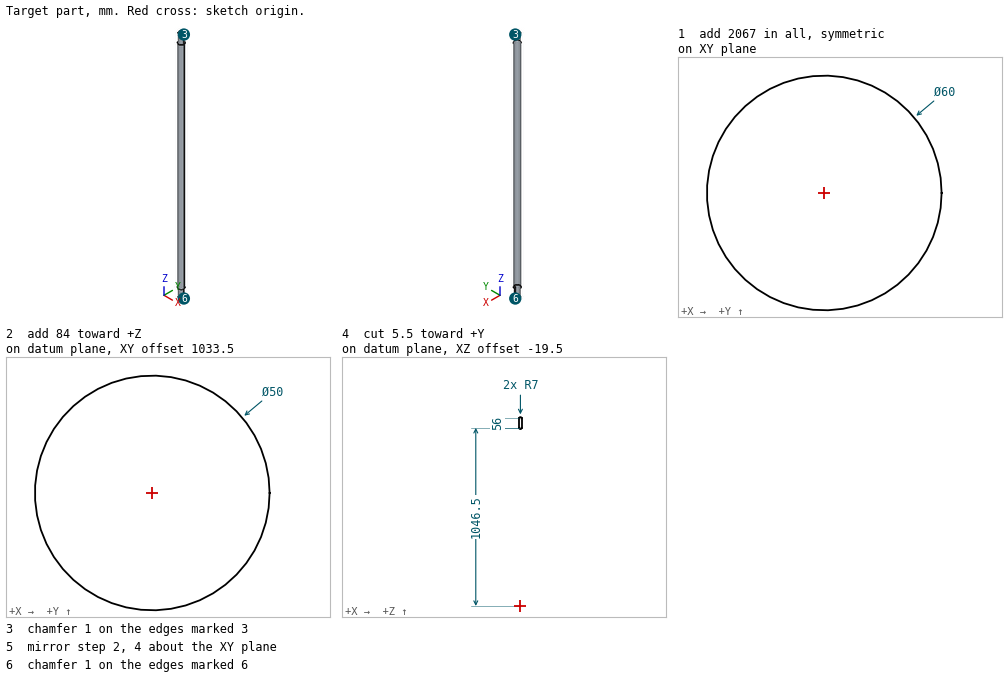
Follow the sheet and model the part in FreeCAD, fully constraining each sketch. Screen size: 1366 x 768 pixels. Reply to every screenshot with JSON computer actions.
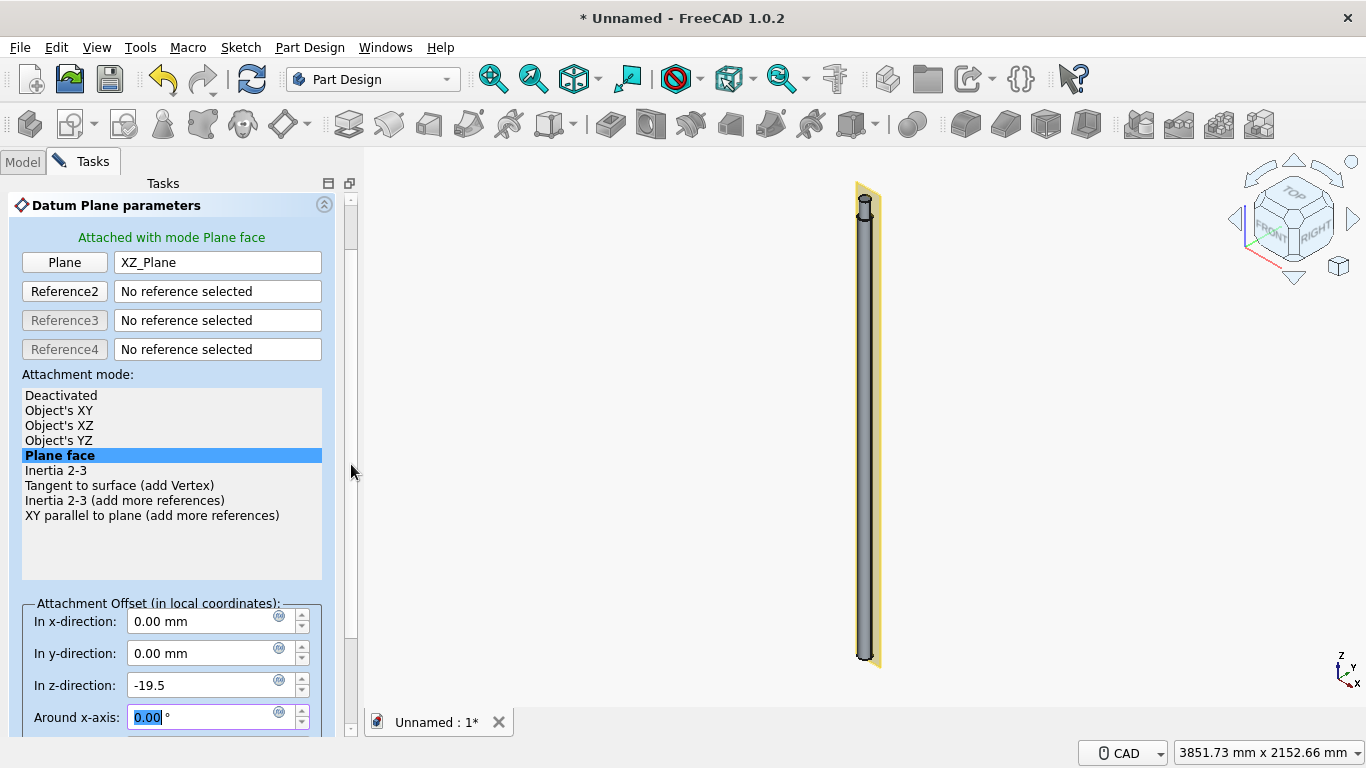
{"action": "left_click", "coordinate": [124, 222]}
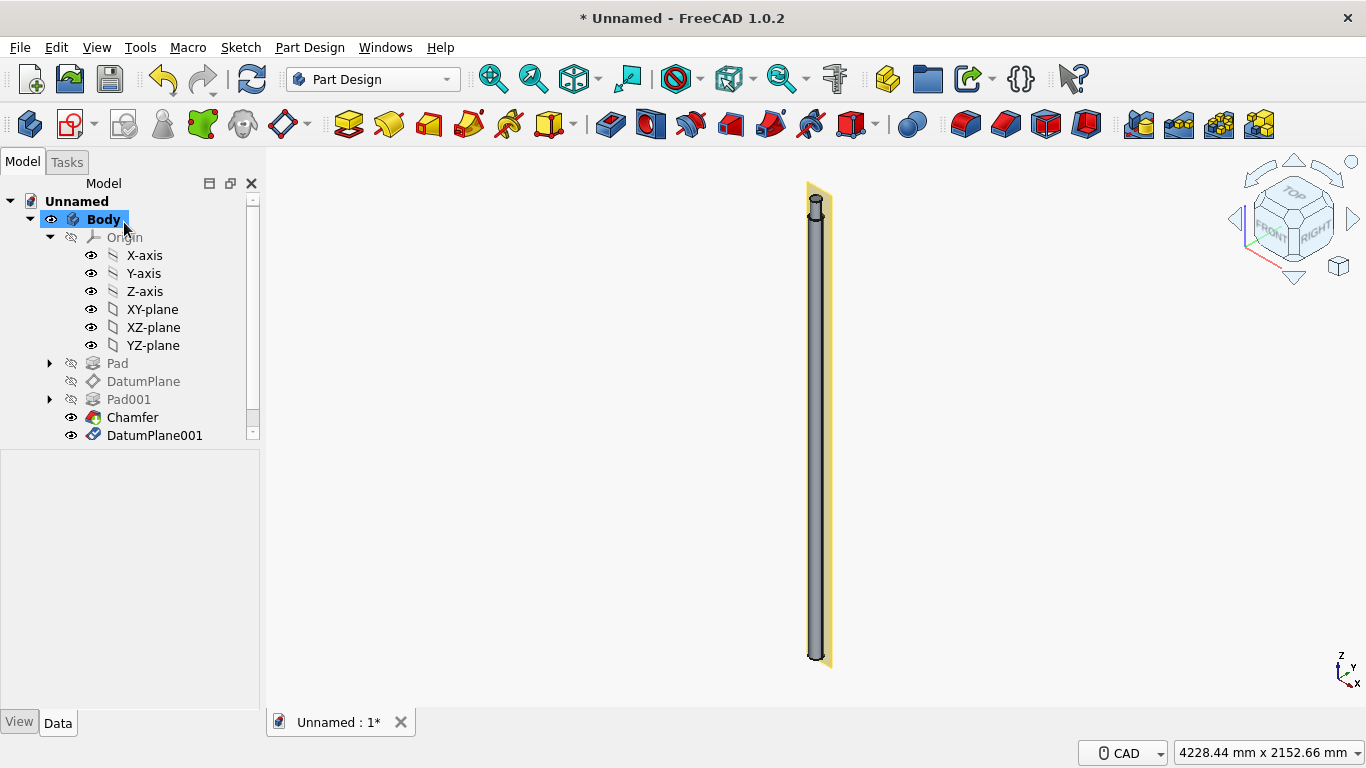
{"action": "left_click", "coordinate": [116, 435]}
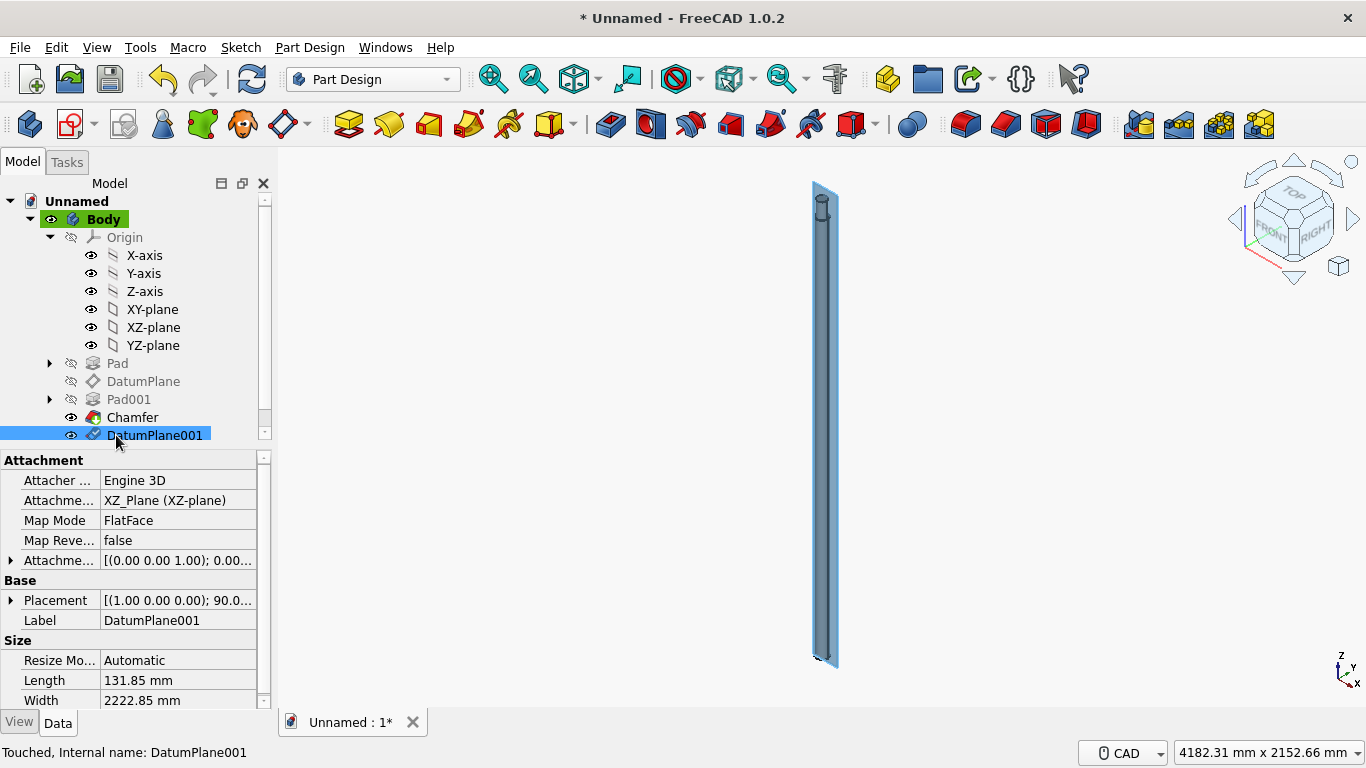
{"action": "left_click", "coordinate": [70, 124]}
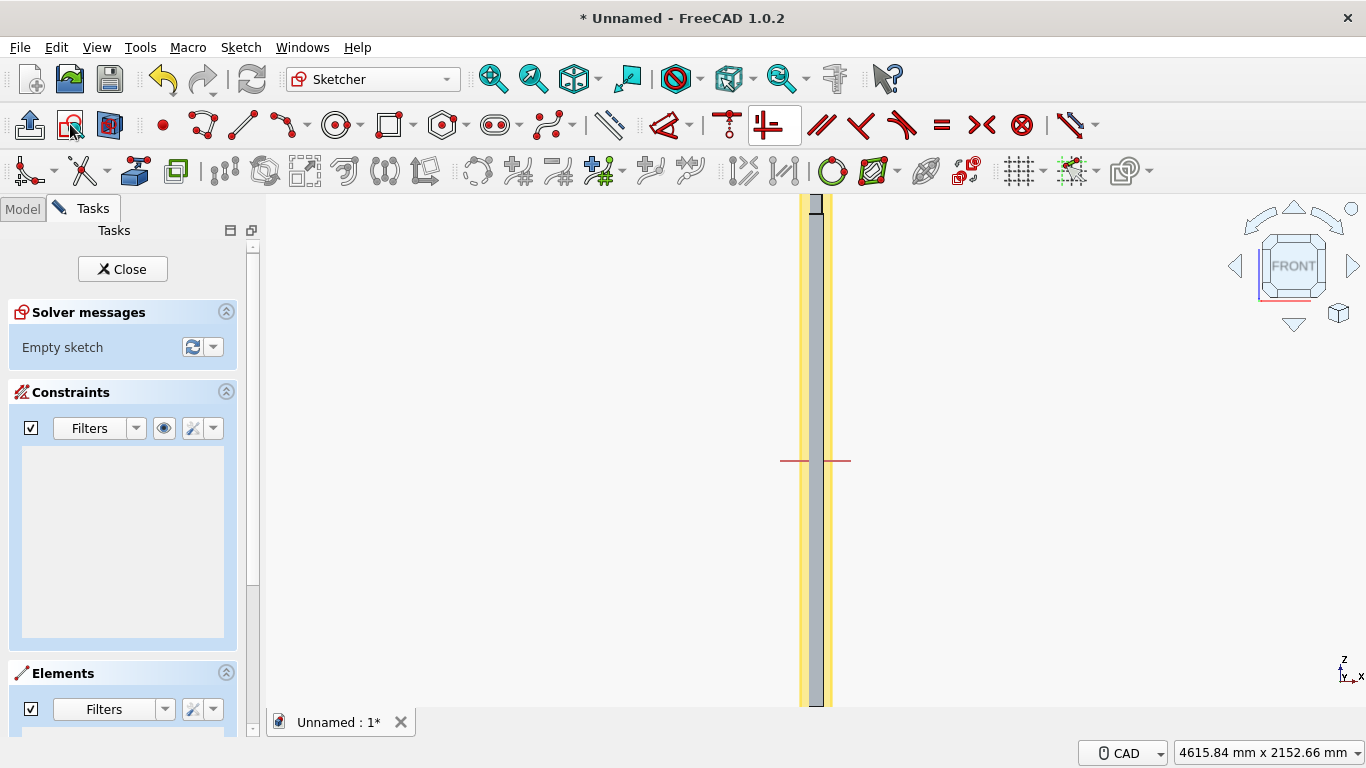
{"action": "left_click", "coordinate": [110, 126]}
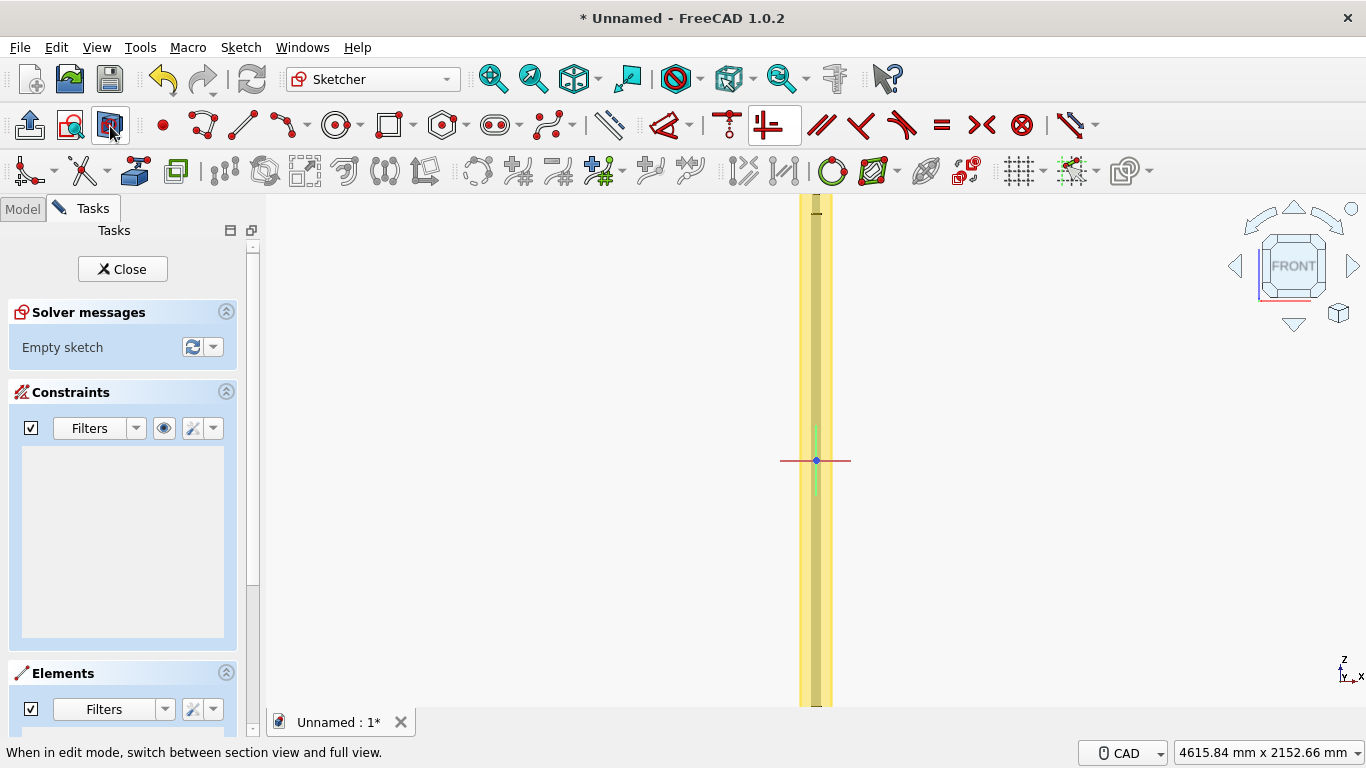
{"action": "scroll", "coordinate": [748, 450], "scroll_direction": "down", "scroll_amount": 5}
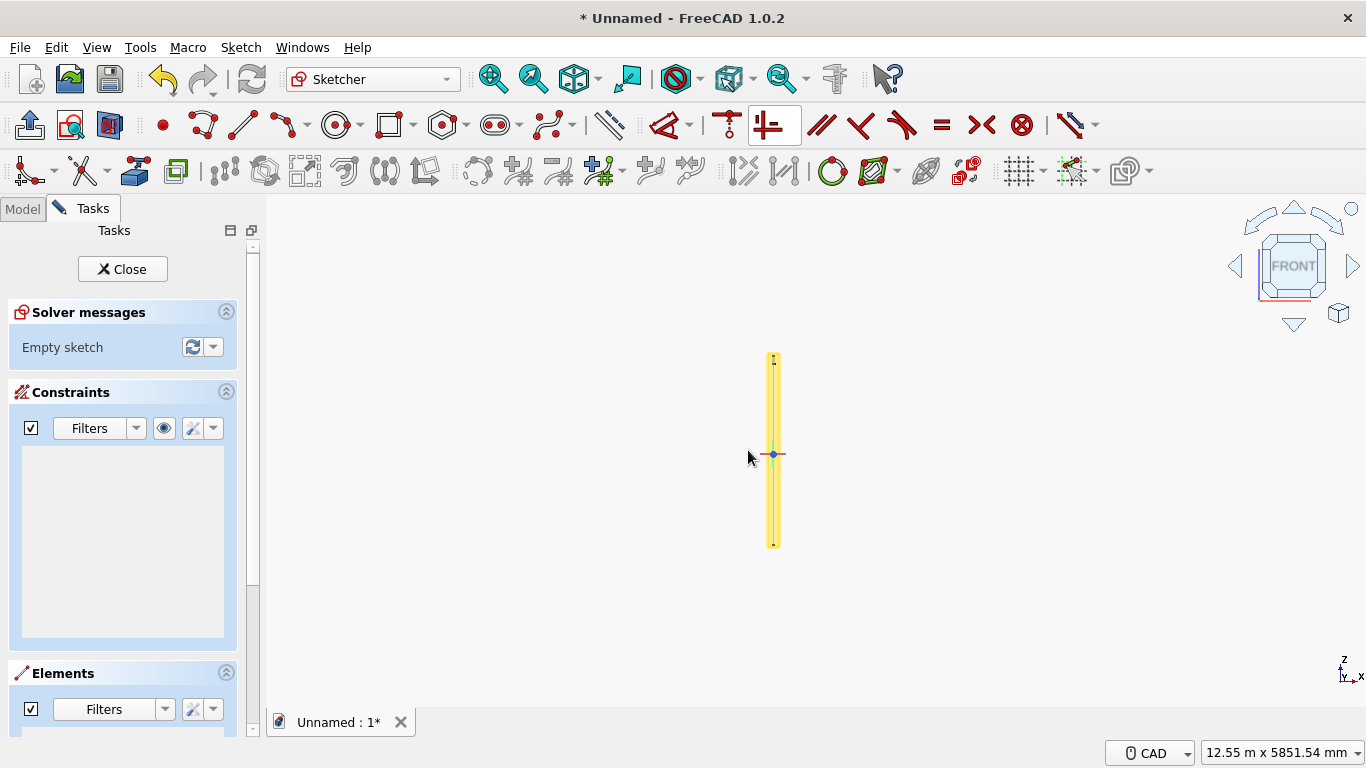
{"action": "scroll", "coordinate": [775, 355], "scroll_direction": "up", "scroll_amount": 15}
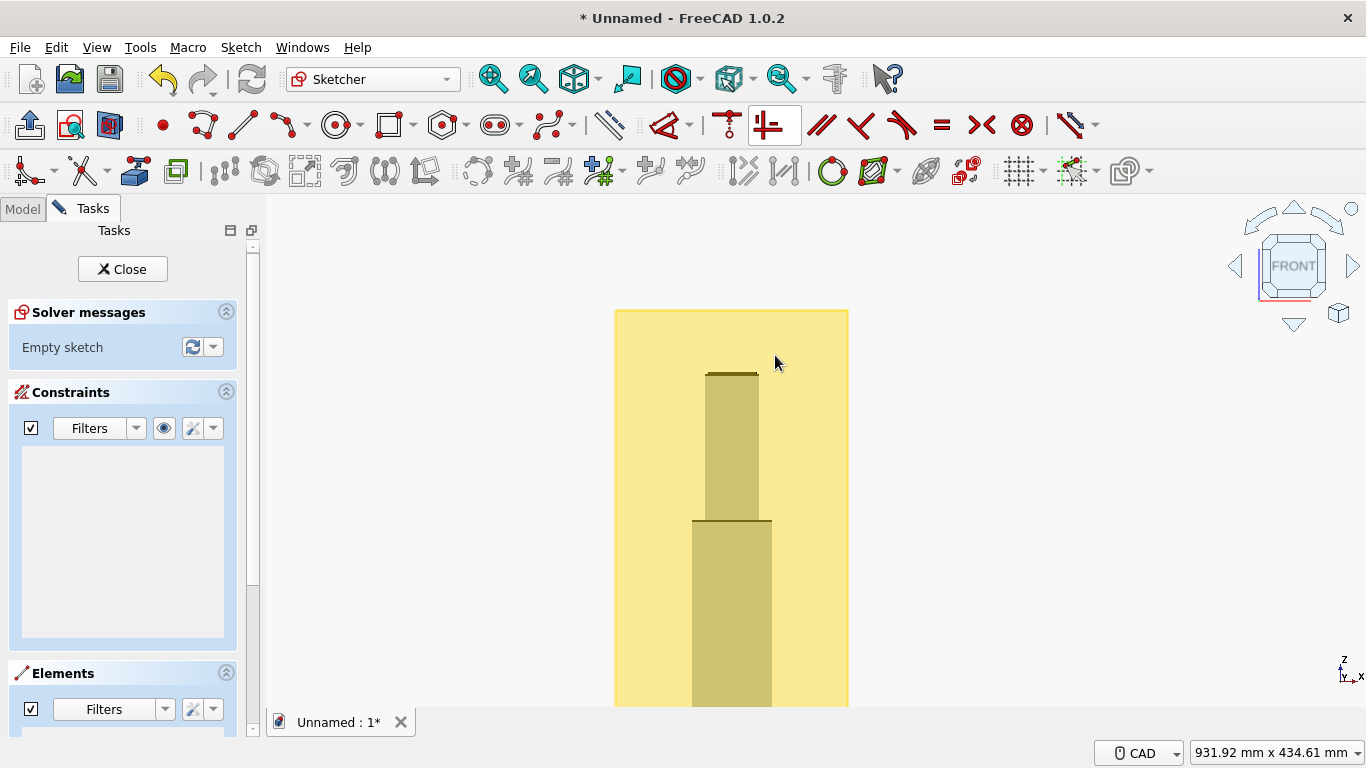
{"action": "scroll", "coordinate": [723, 448], "scroll_direction": "up", "scroll_amount": 5}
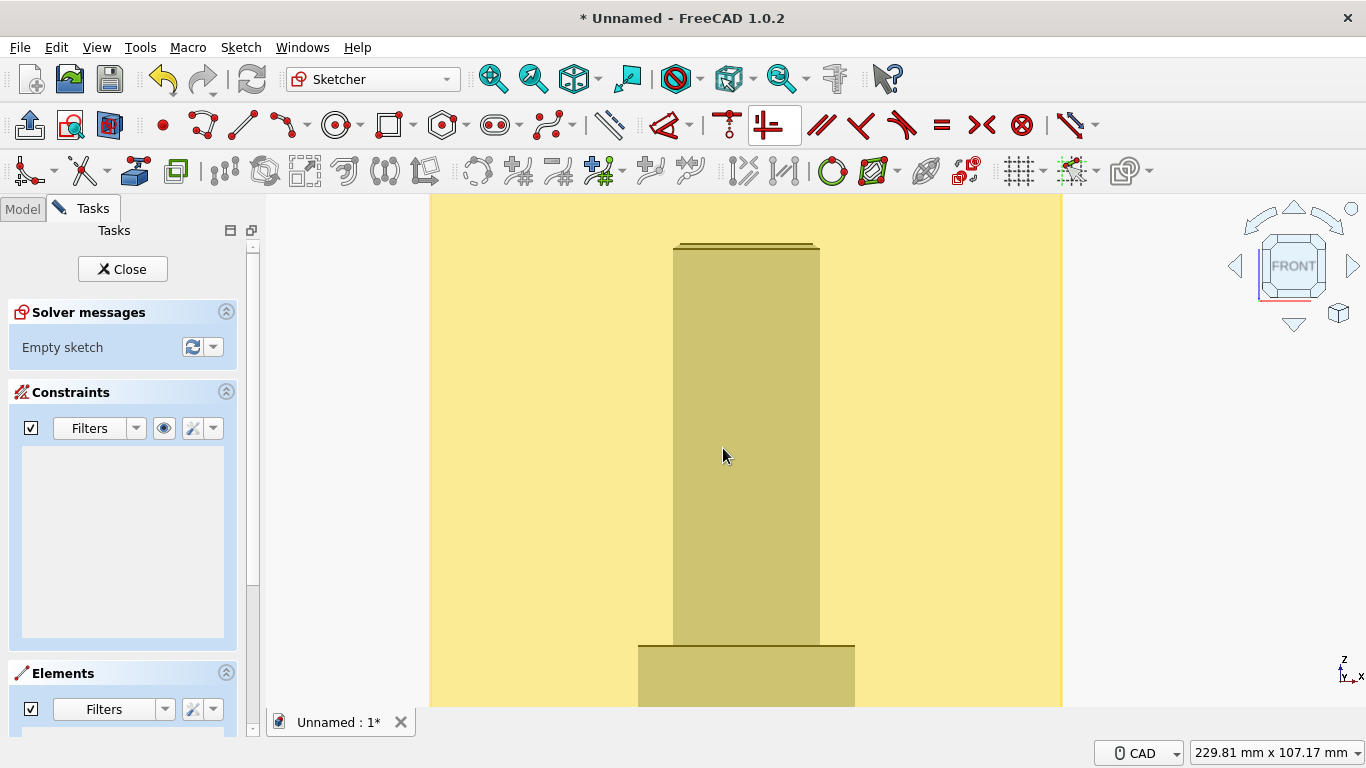
{"action": "left_click", "coordinate": [496, 126]}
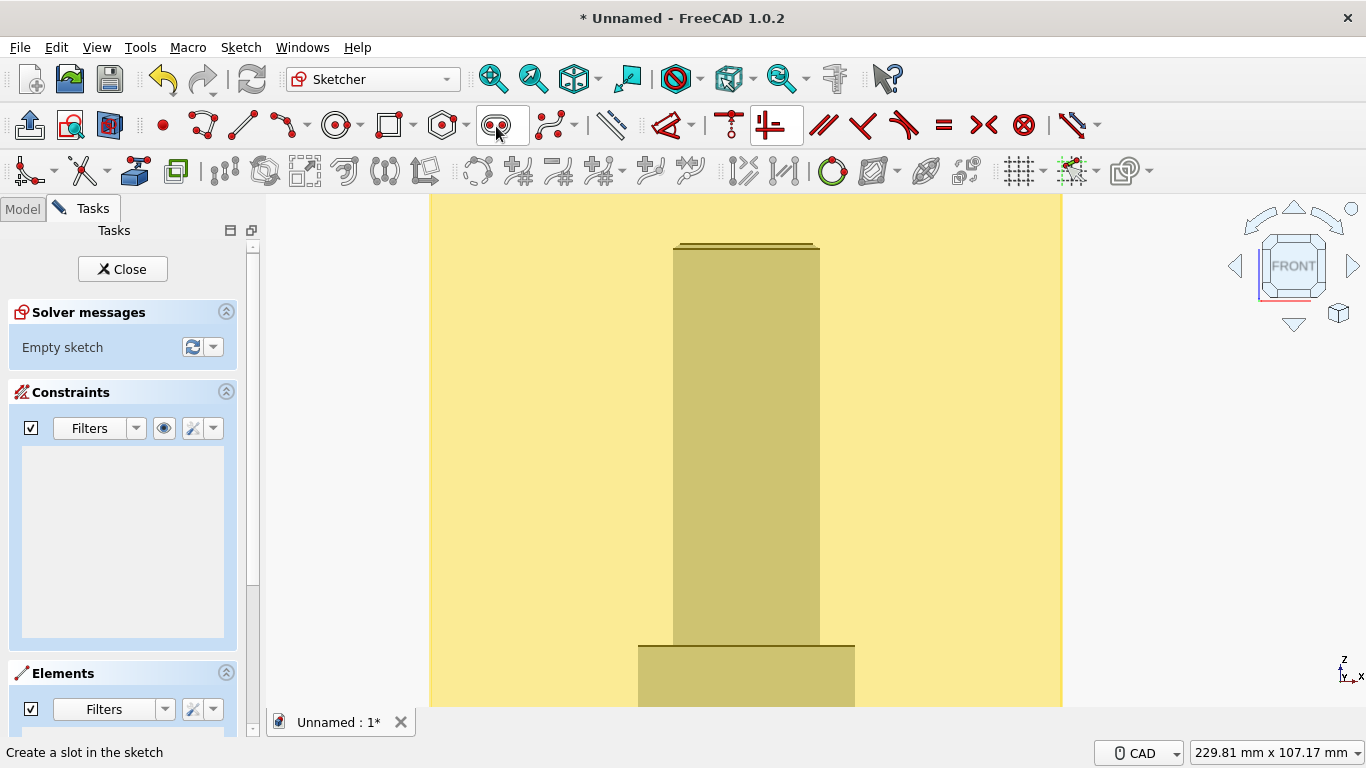
{"action": "left_click", "coordinate": [746, 584]}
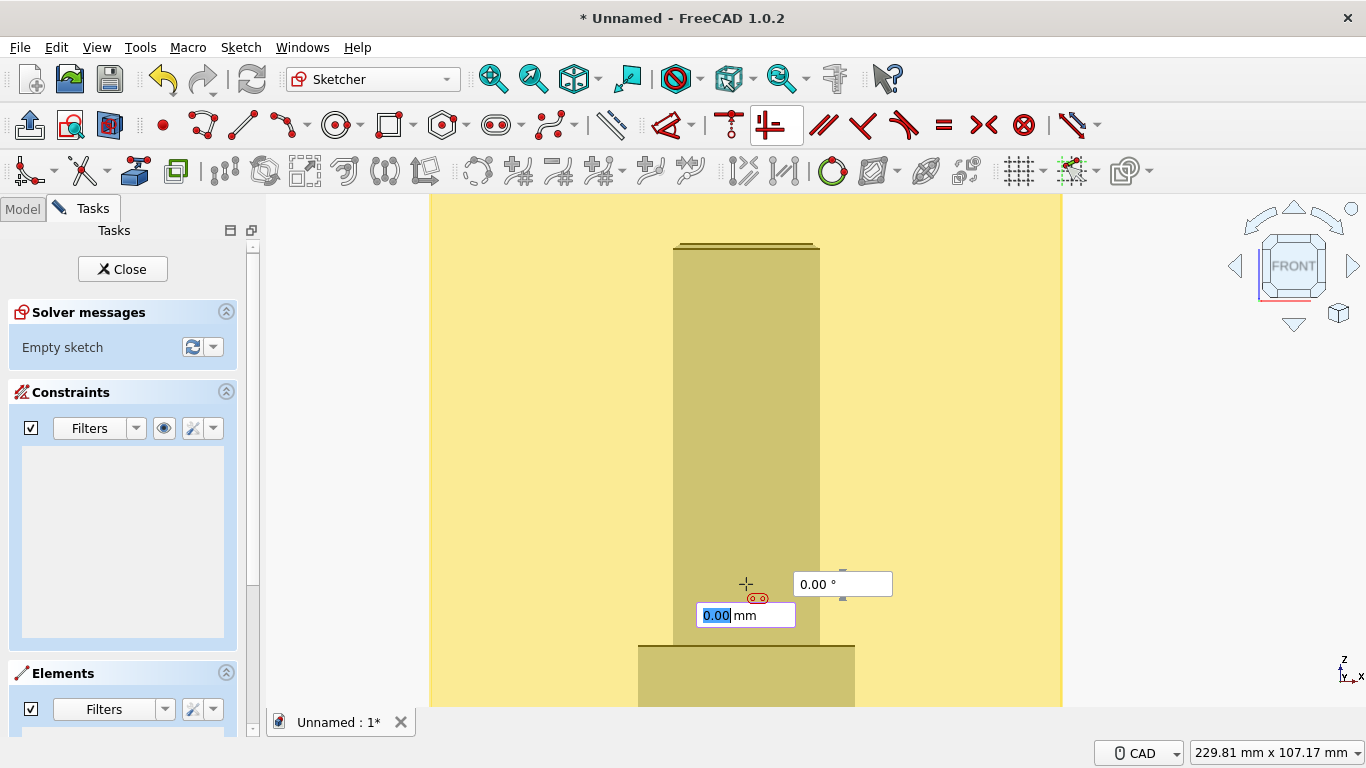
{"action": "left_click", "coordinate": [755, 316]}